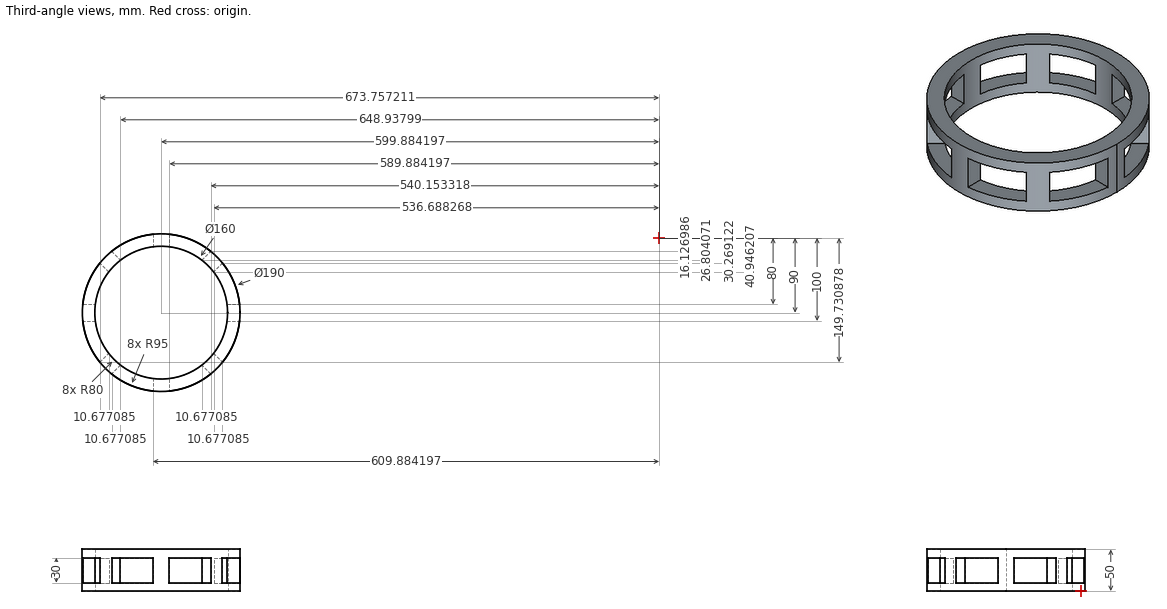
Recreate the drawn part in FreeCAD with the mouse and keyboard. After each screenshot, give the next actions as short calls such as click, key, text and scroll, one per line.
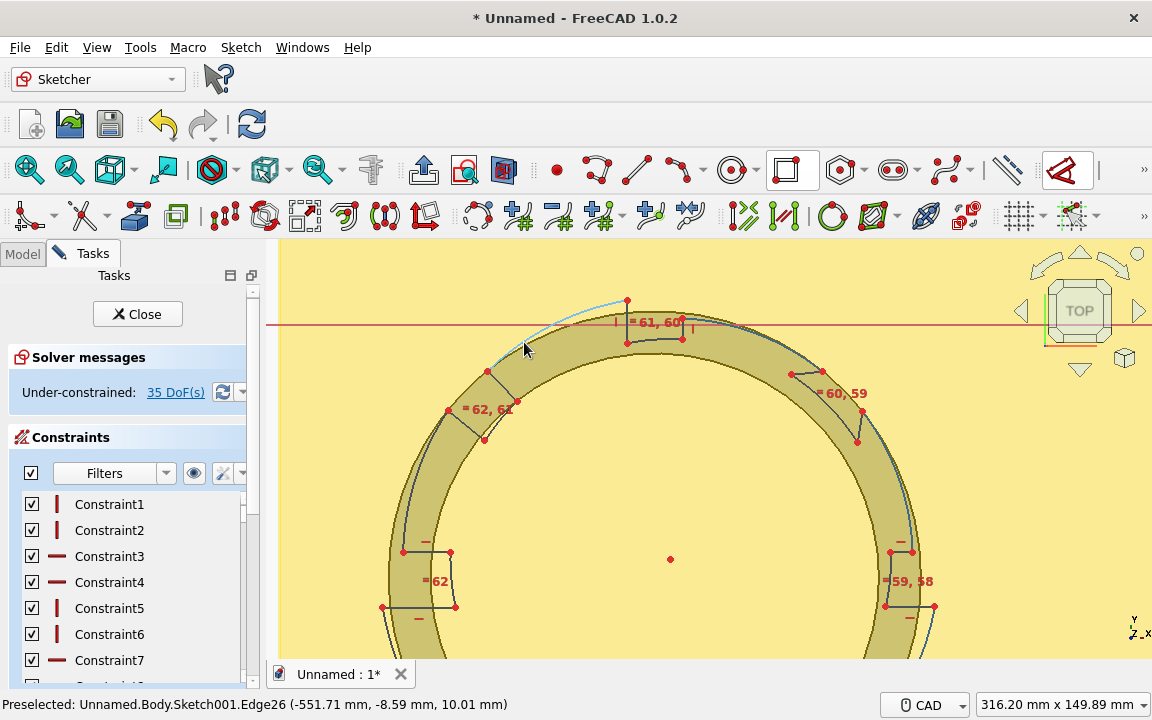
click(525, 341)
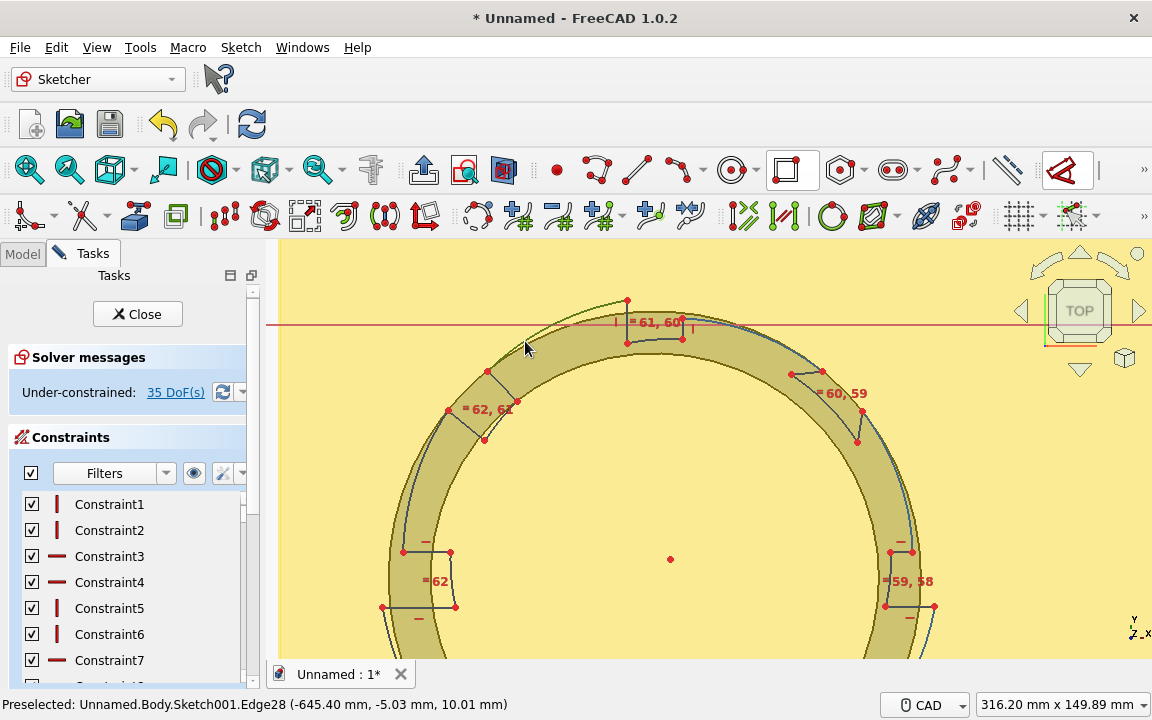
click(426, 450)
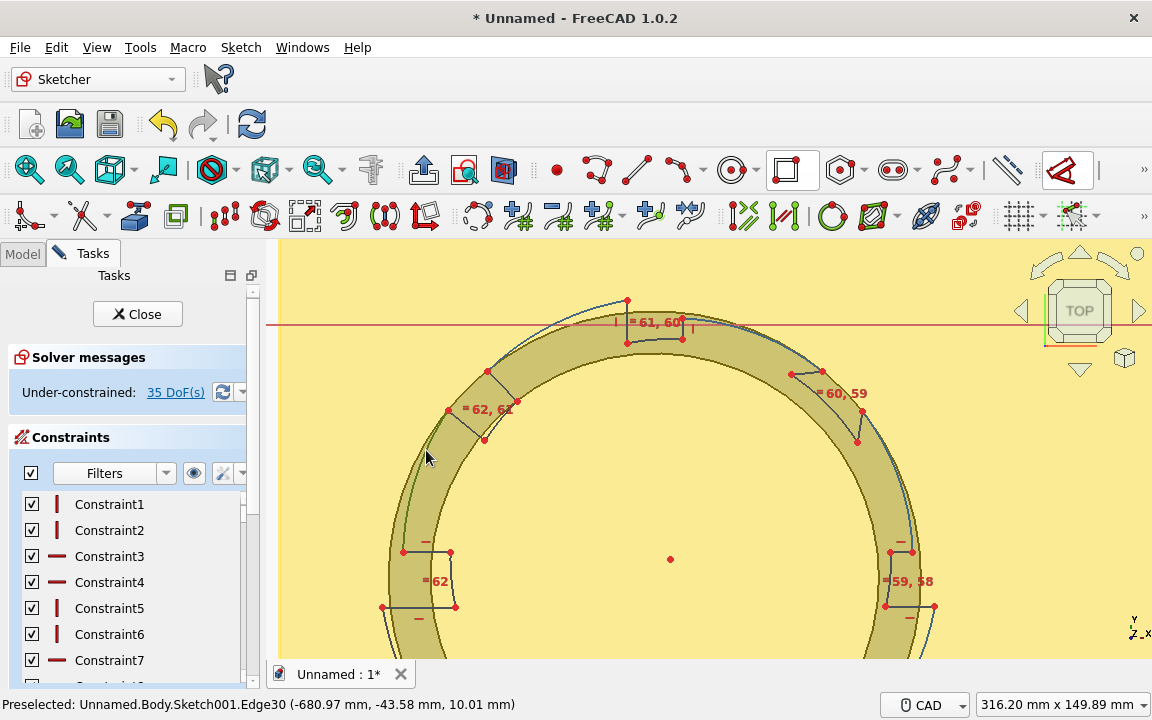
scroll(629, 344, down, 4)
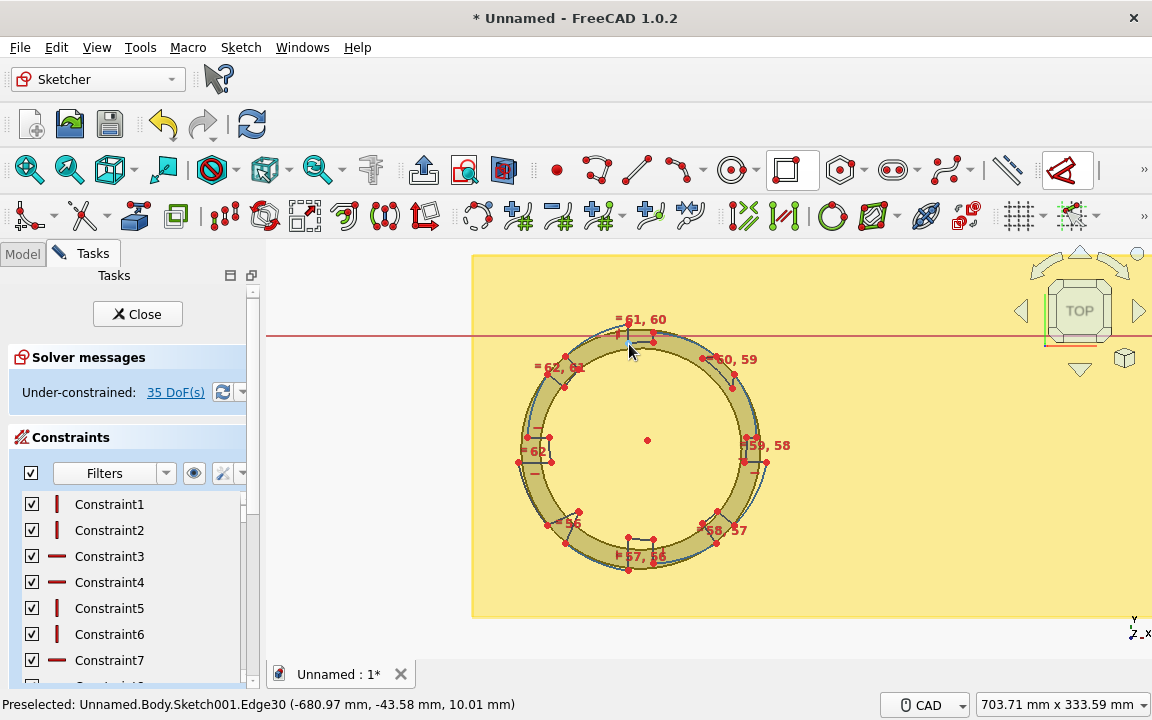
click(524, 483)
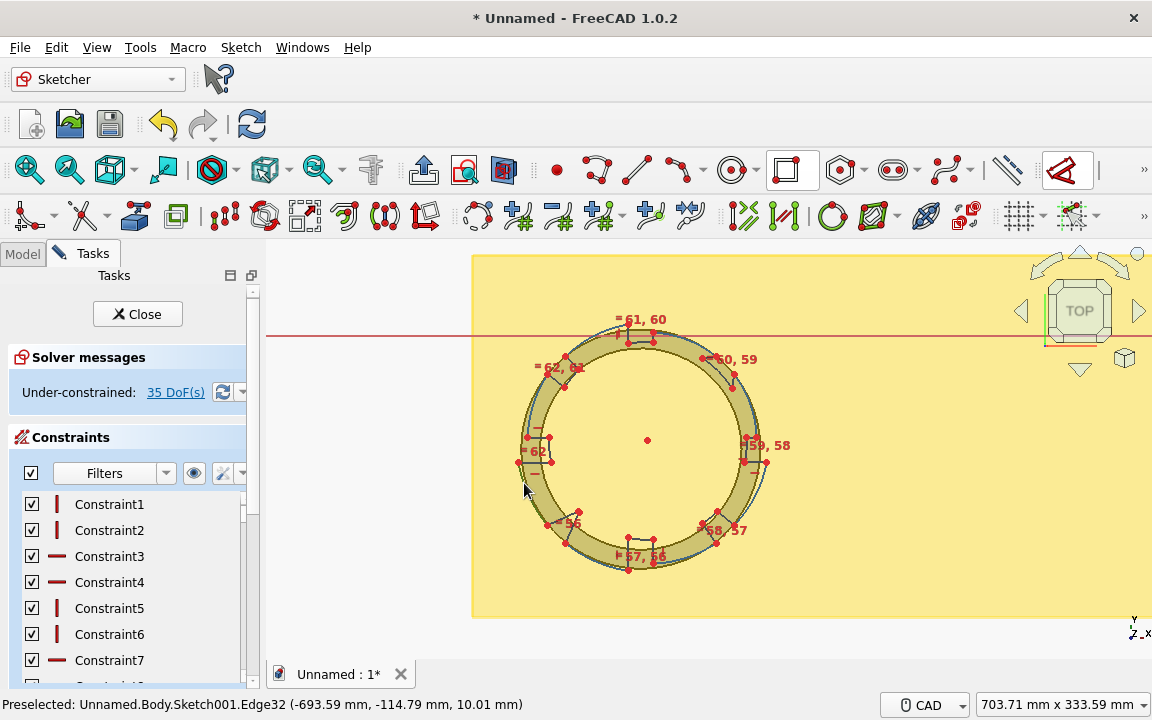
key(e)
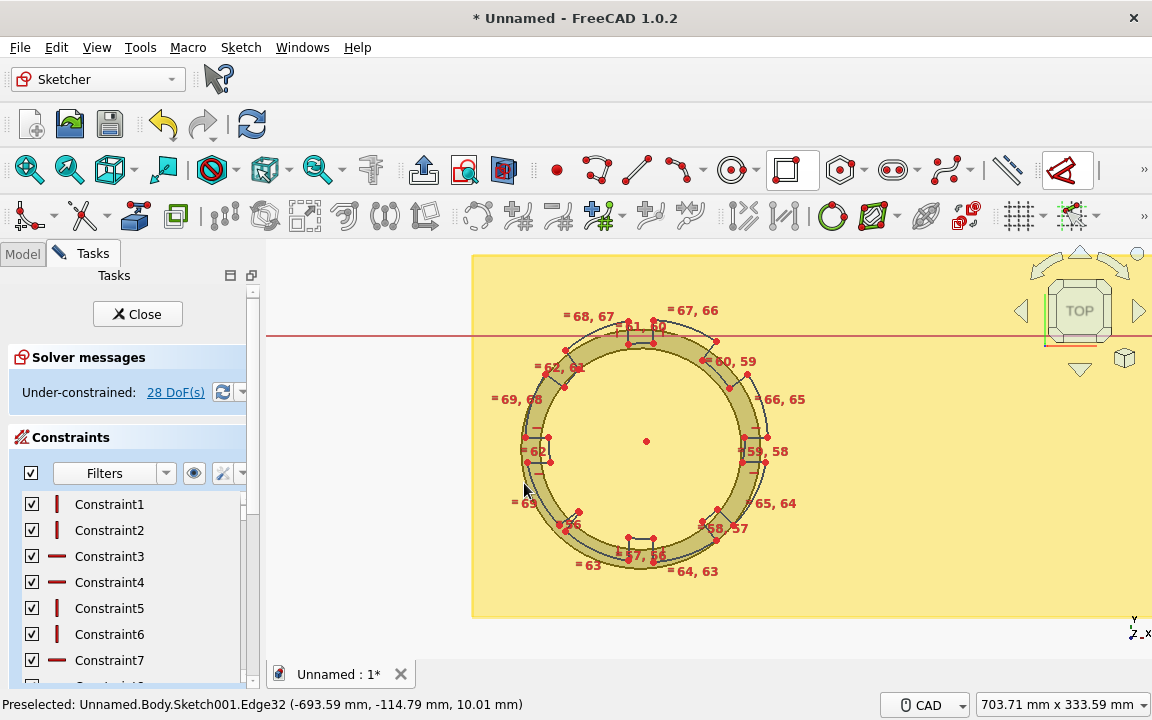
scroll(579, 512, up, 15)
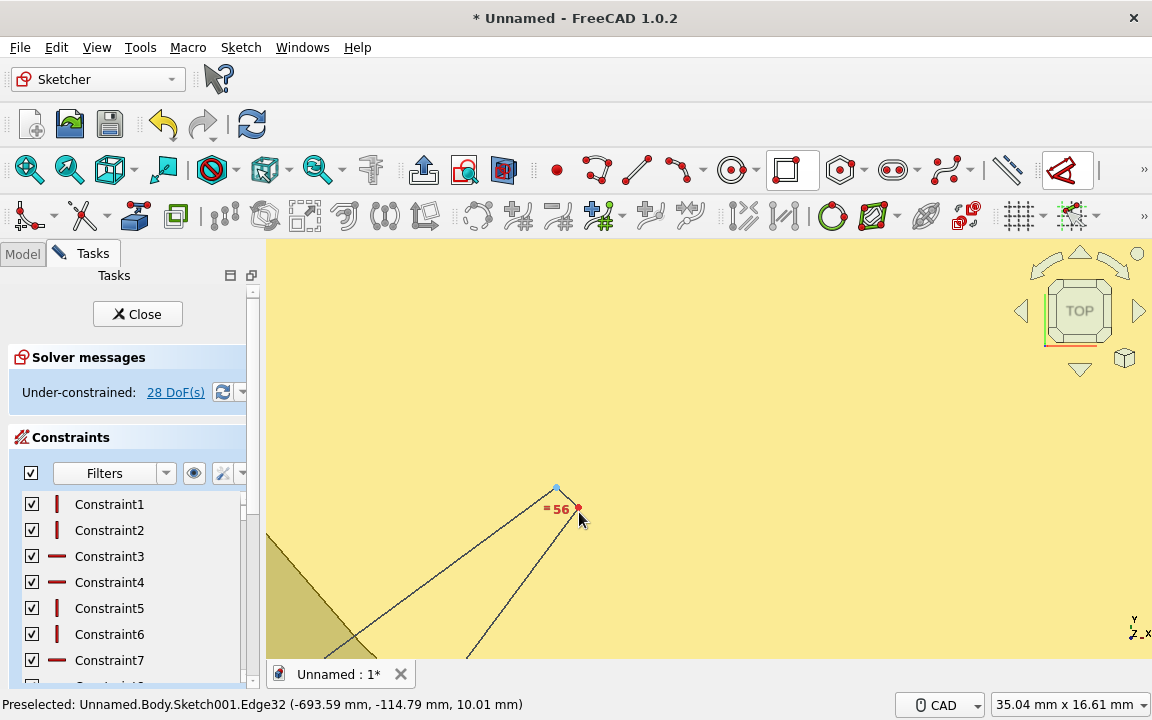
click(567, 498)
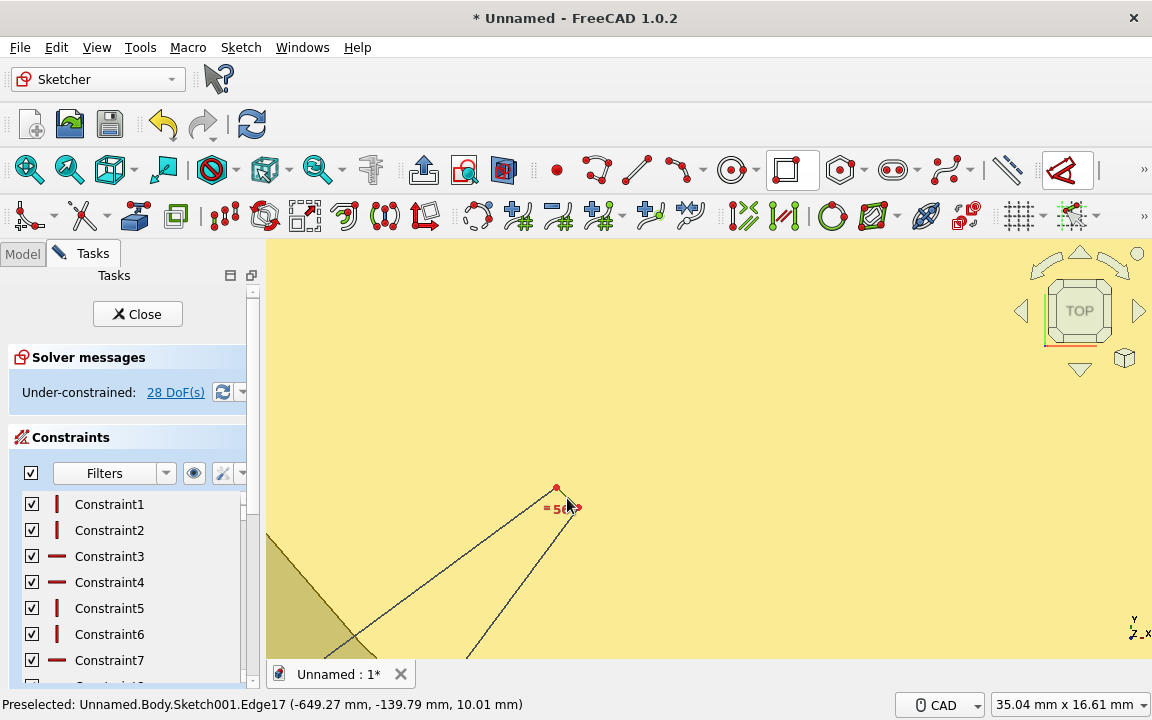
key(k)
key(r)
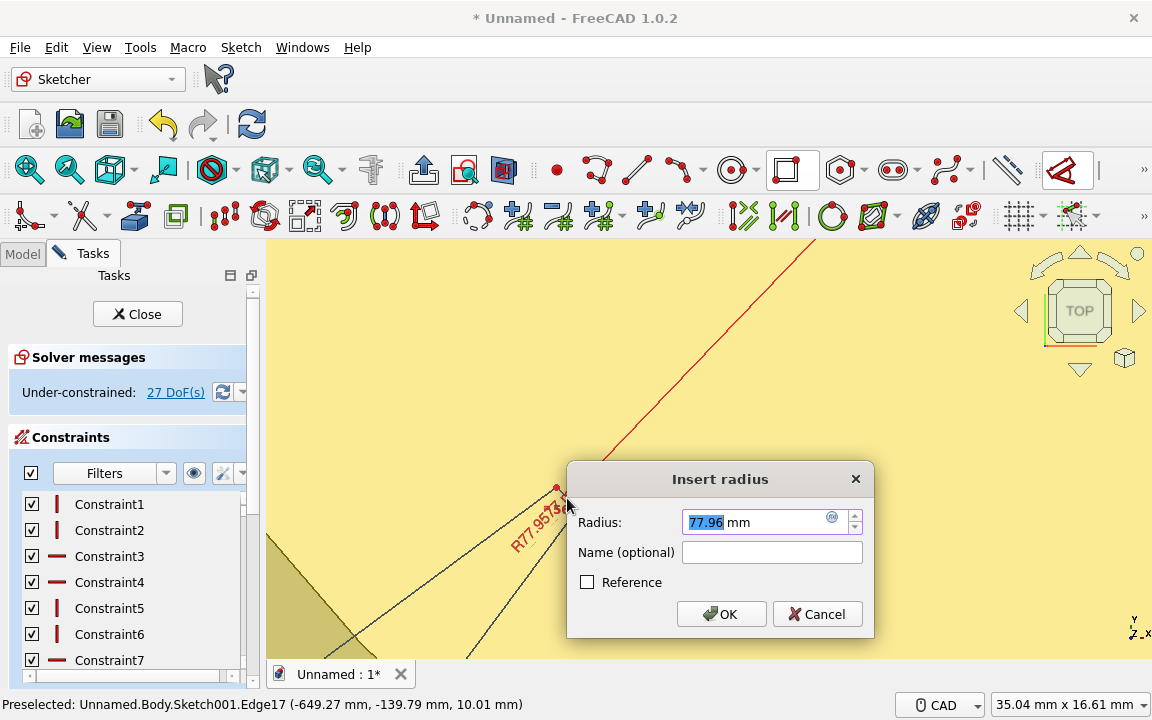
text(80)
key(Return)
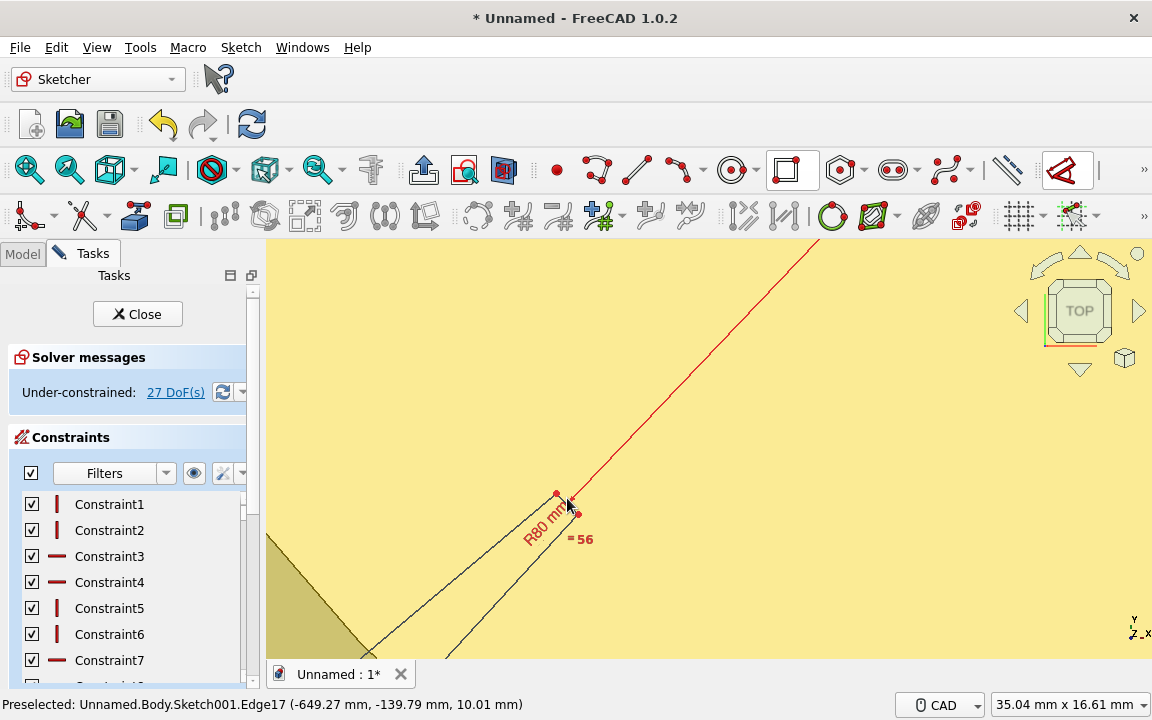
scroll(579, 513, down, 15)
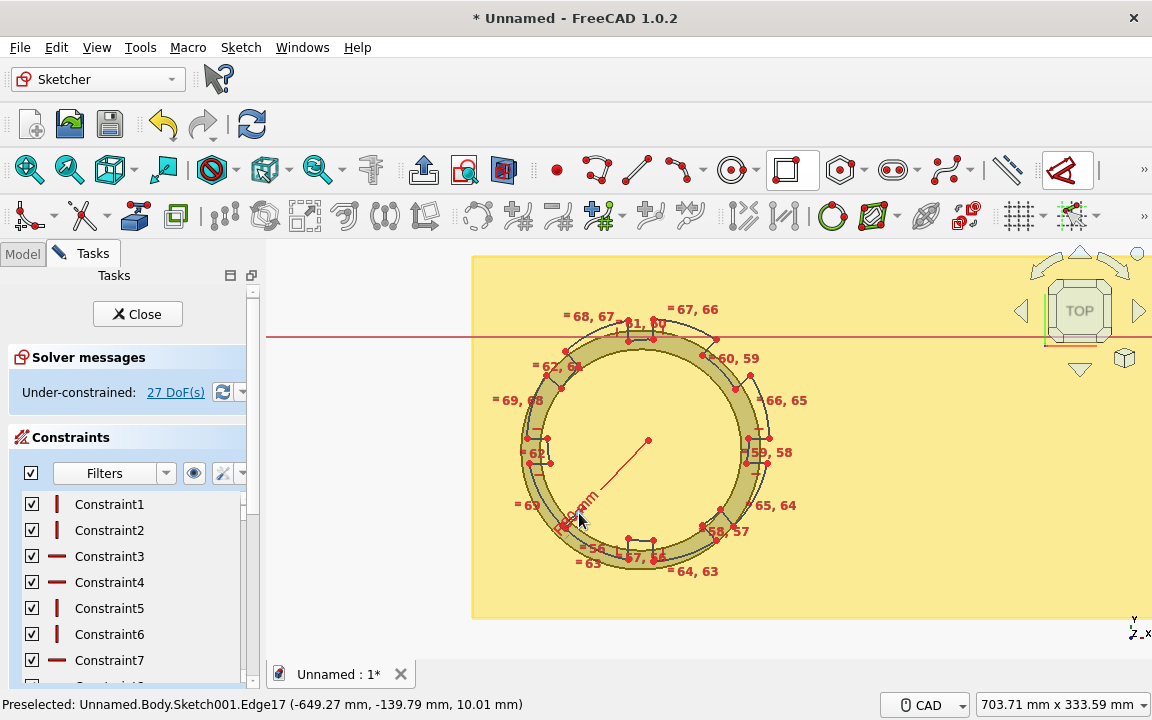
click(608, 554)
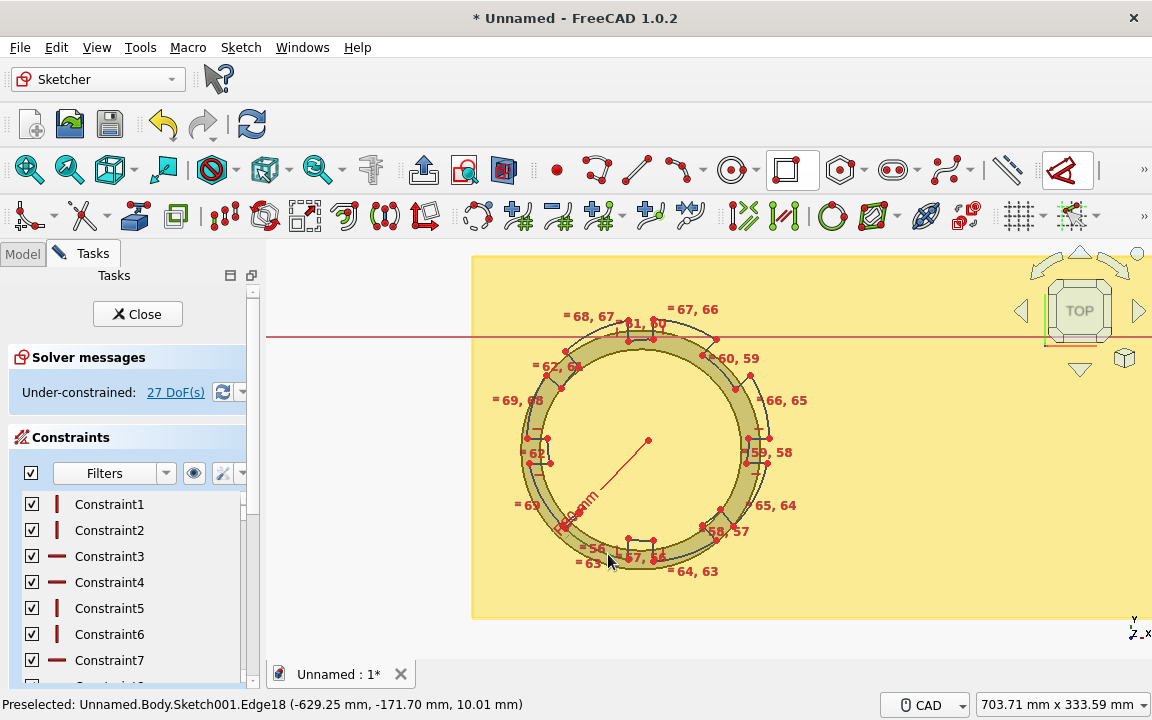
key(k)
key(r)